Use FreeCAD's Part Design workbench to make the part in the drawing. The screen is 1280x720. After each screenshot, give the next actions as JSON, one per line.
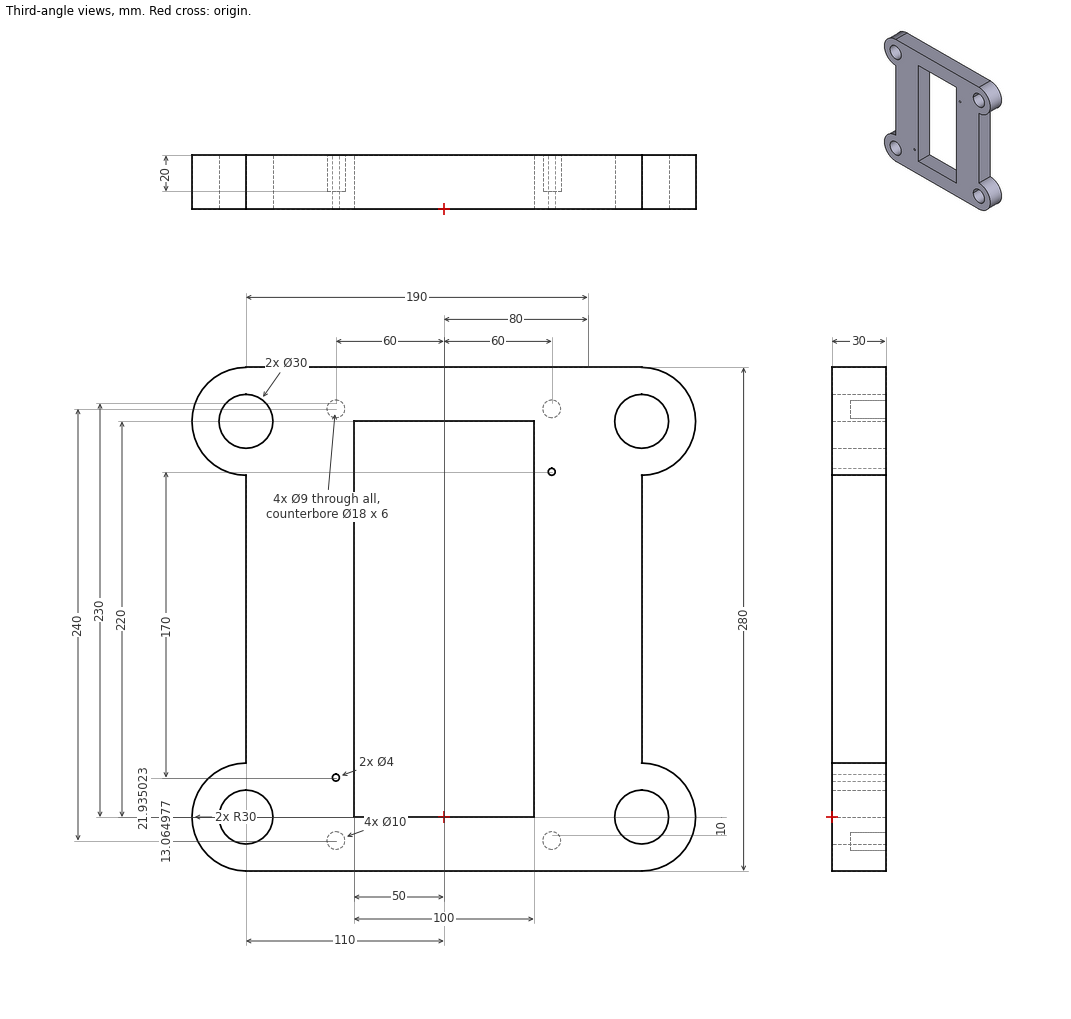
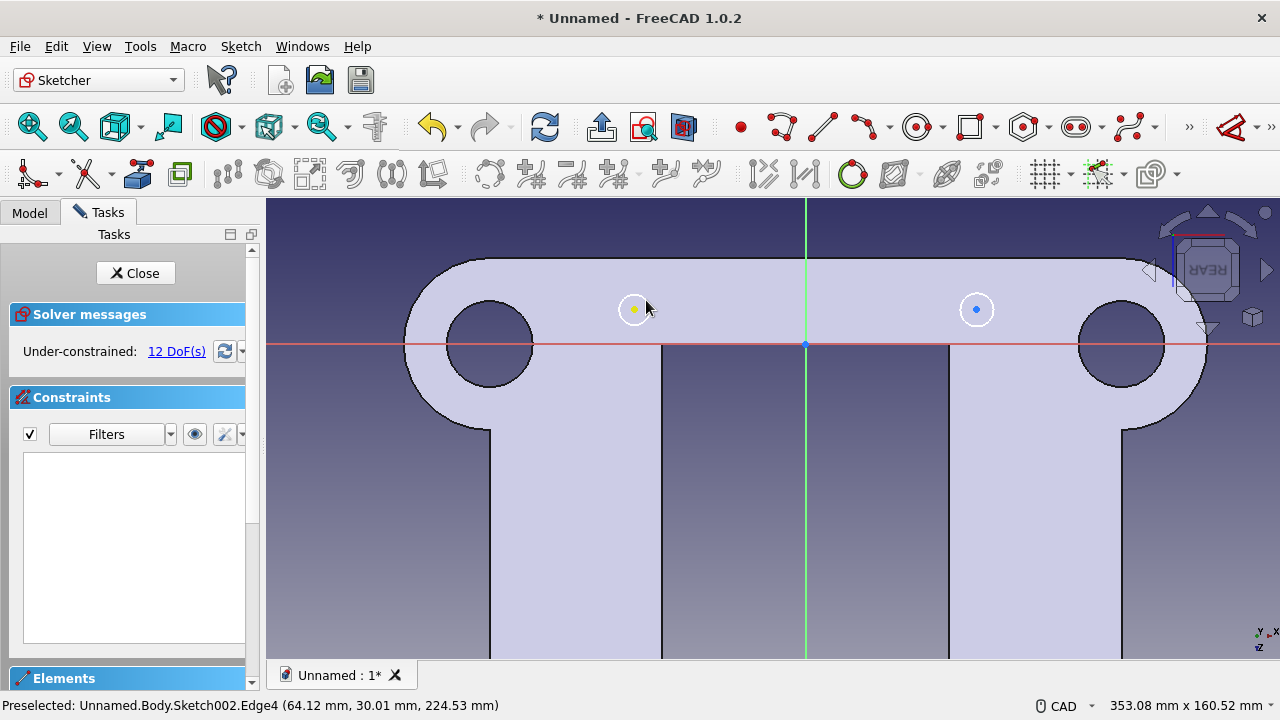
{"action": "left_click", "coordinate": [645, 299]}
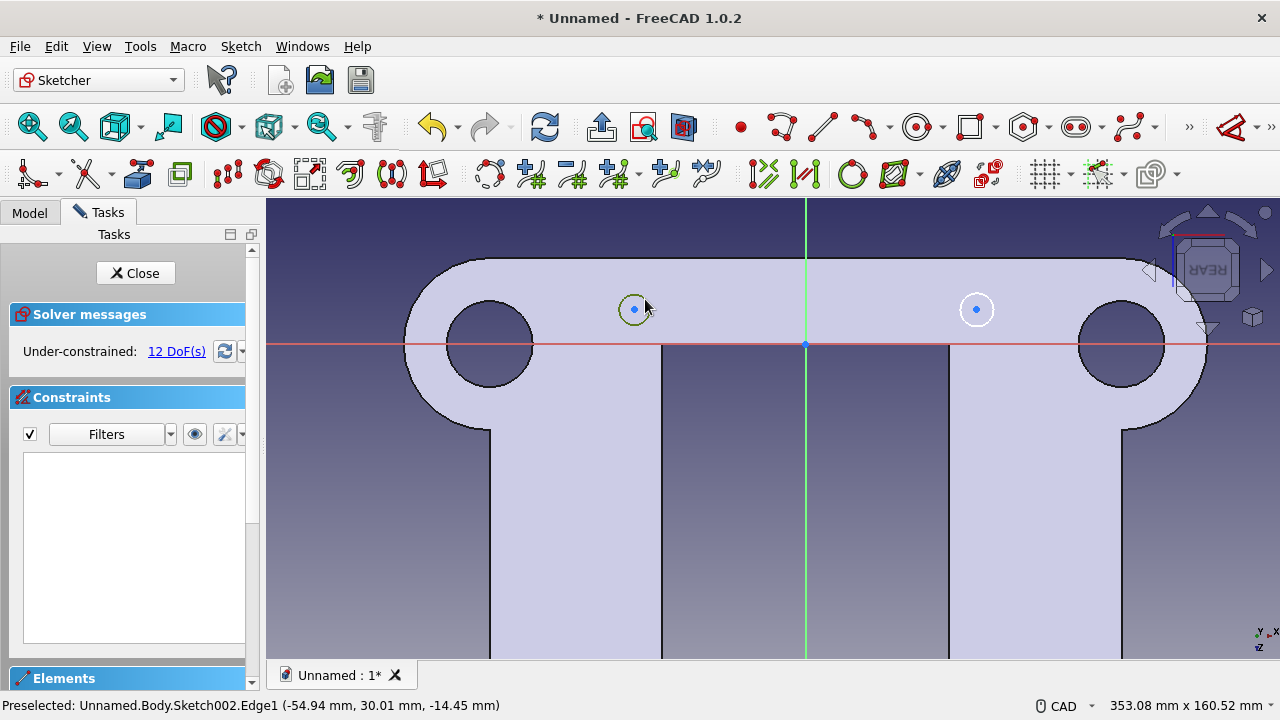
{"action": "scroll", "coordinate": [646, 299], "scroll_direction": "down", "scroll_amount": 5}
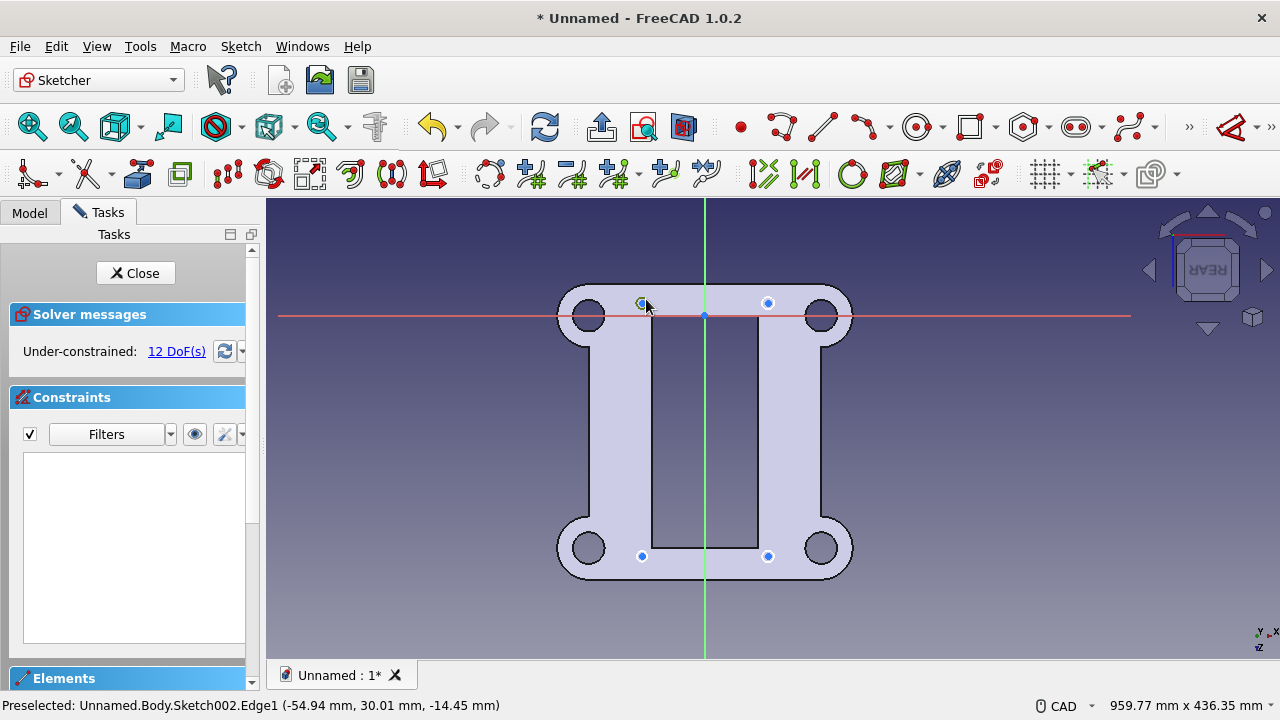
{"action": "scroll", "coordinate": [646, 553], "scroll_direction": "up", "scroll_amount": 5}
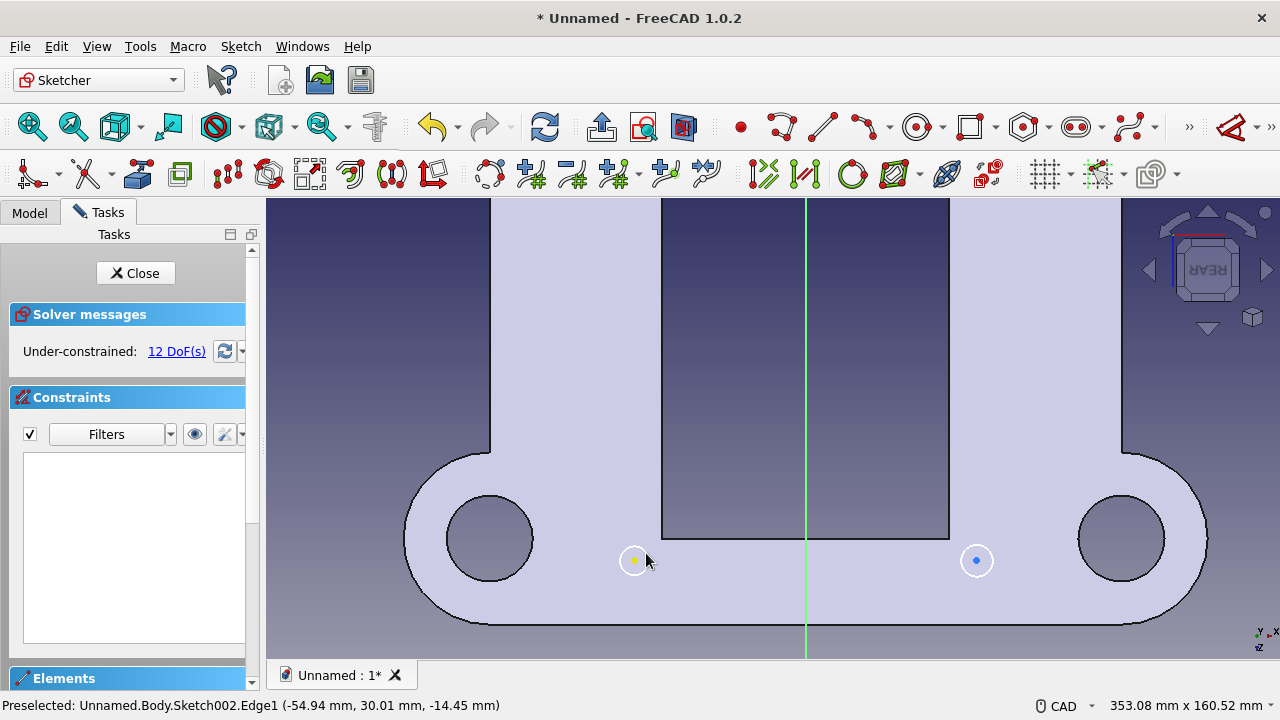
{"action": "left_click", "coordinate": [645, 551]}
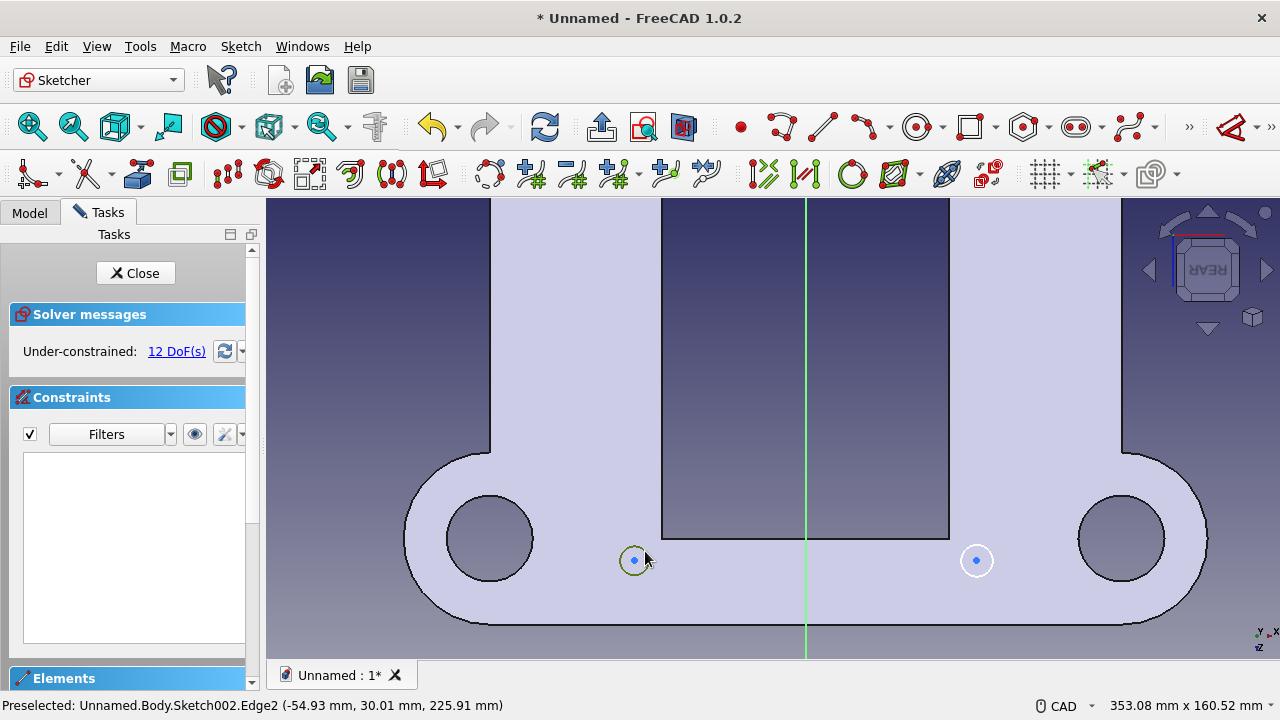
{"action": "scroll", "coordinate": [646, 553], "scroll_direction": "down", "scroll_amount": 5}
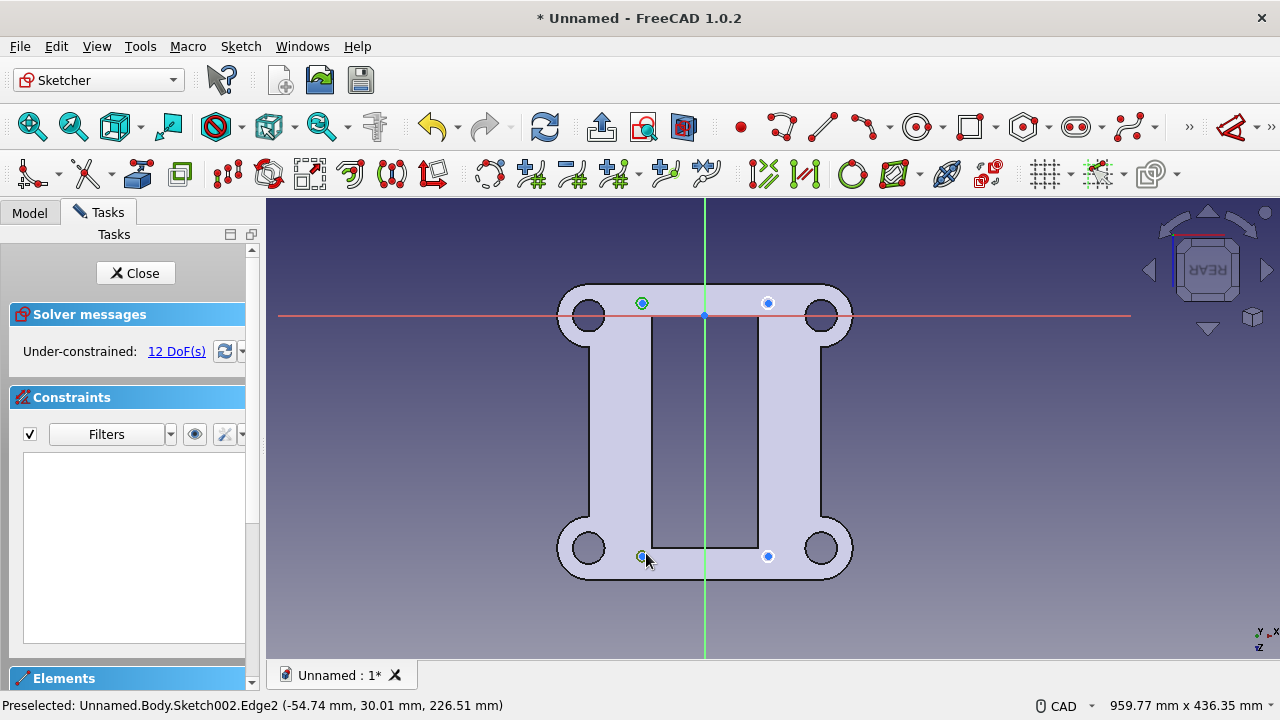
{"action": "scroll", "coordinate": [772, 299], "scroll_direction": "up", "scroll_amount": 5}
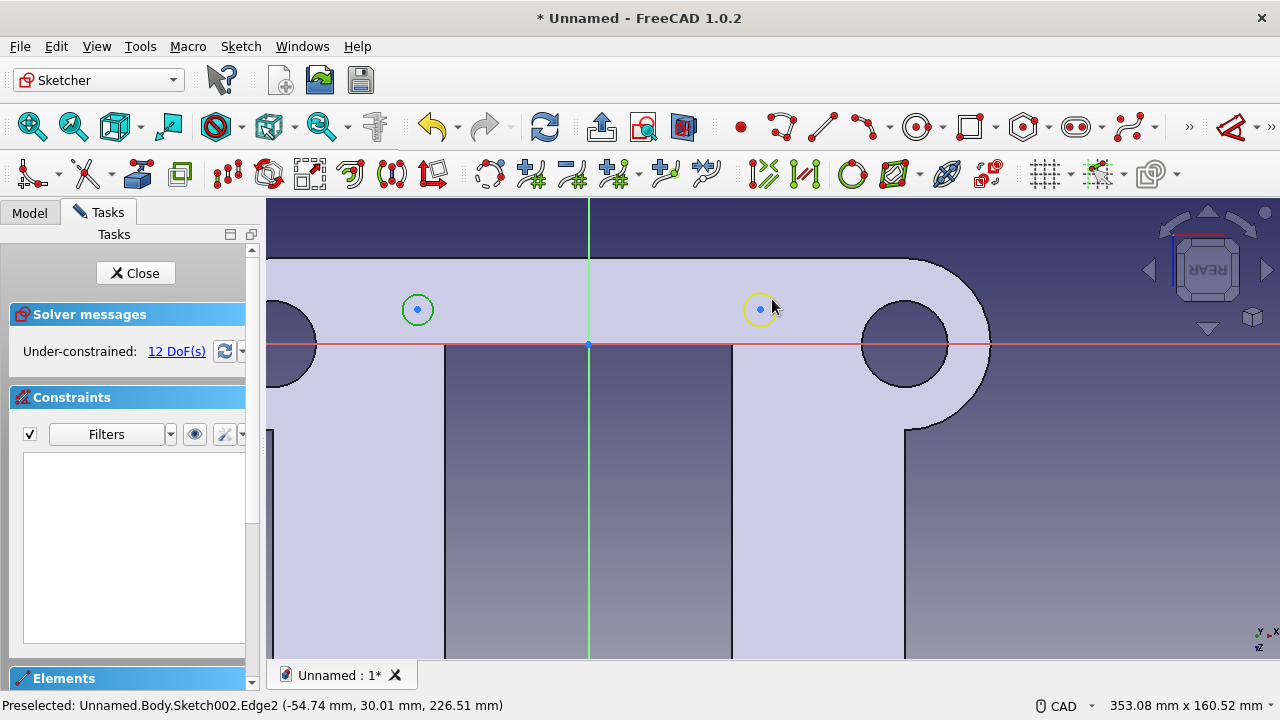
{"action": "left_click", "coordinate": [772, 298]}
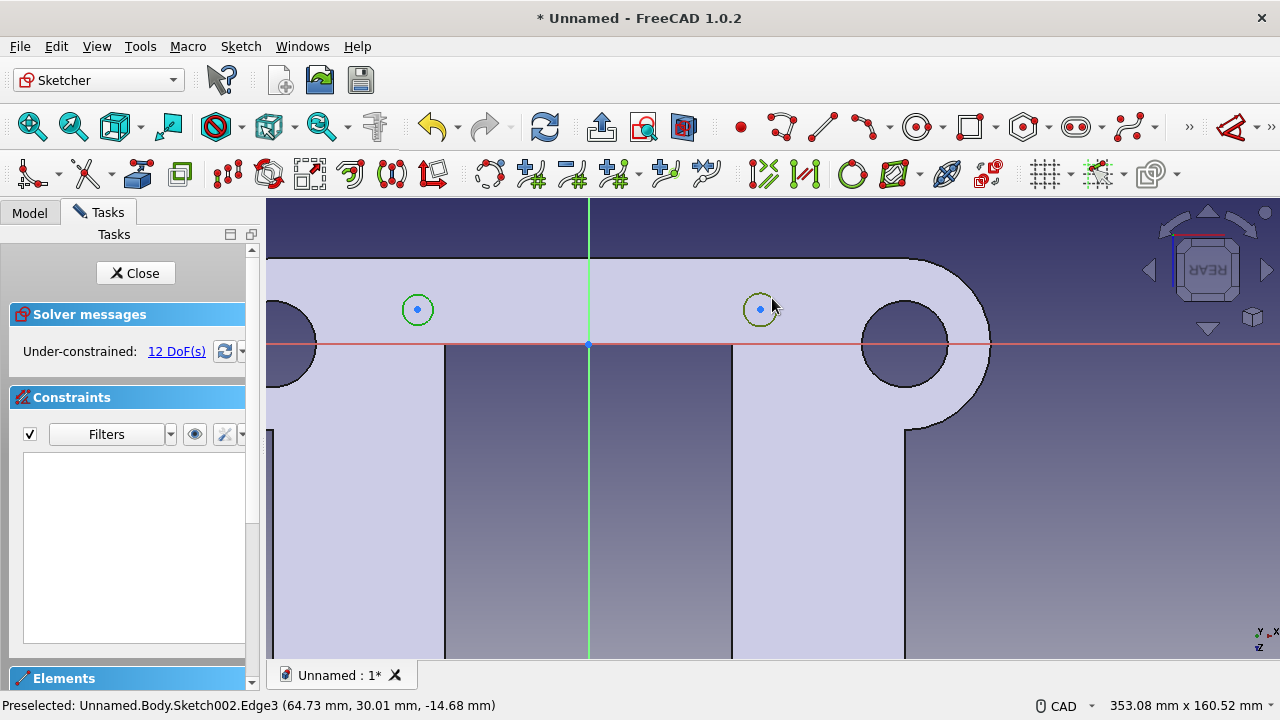
{"action": "scroll", "coordinate": [772, 299], "scroll_direction": "down", "scroll_amount": 5}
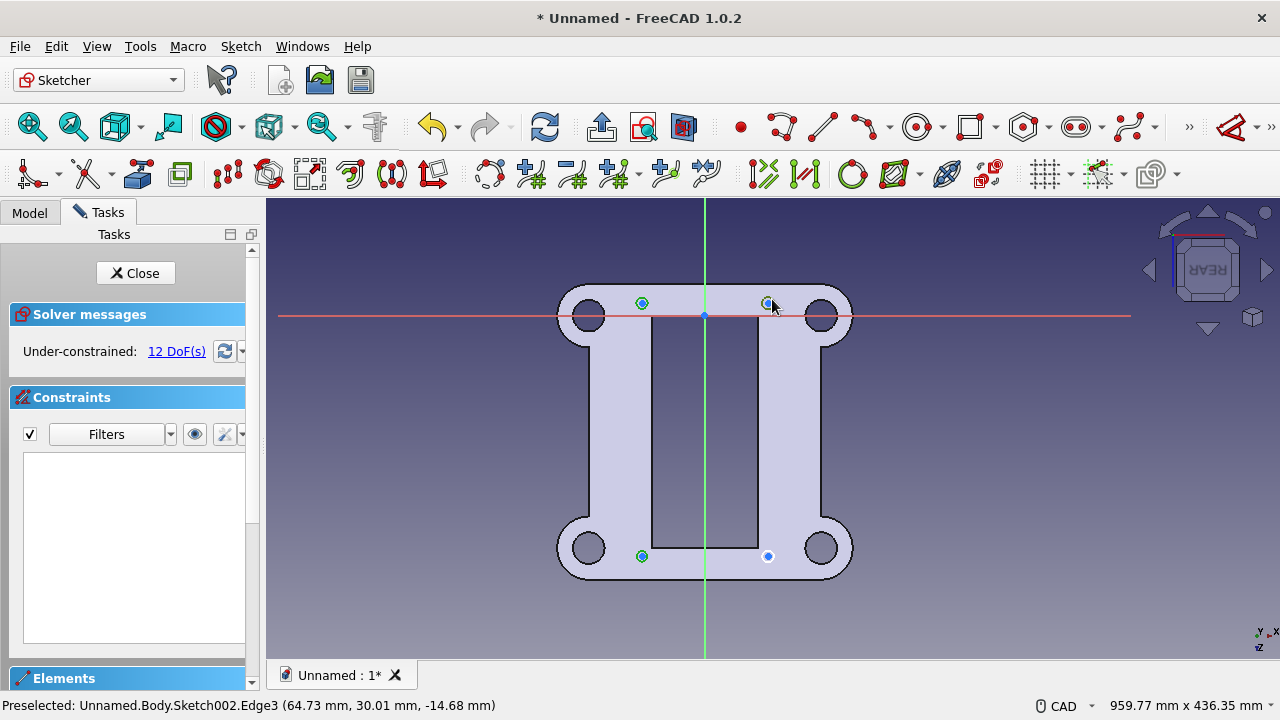
{"action": "scroll", "coordinate": [772, 552], "scroll_direction": "up", "scroll_amount": 5}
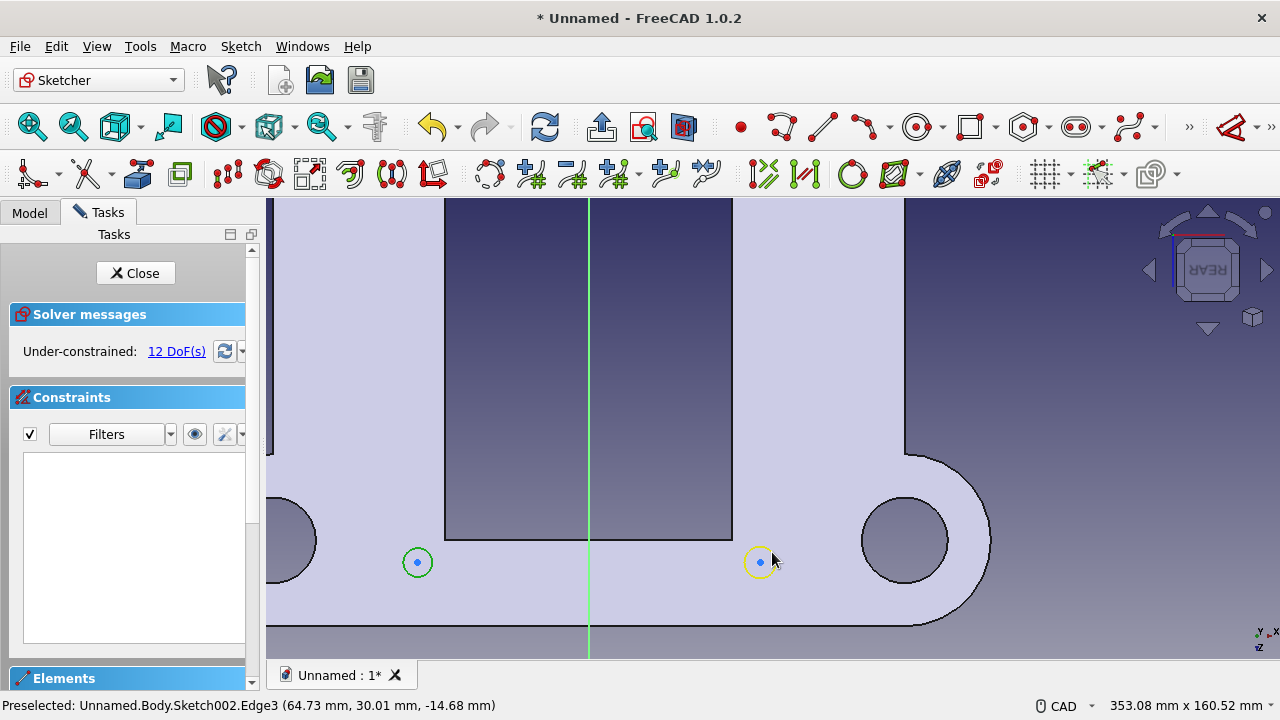
{"action": "left_click", "coordinate": [771, 551]}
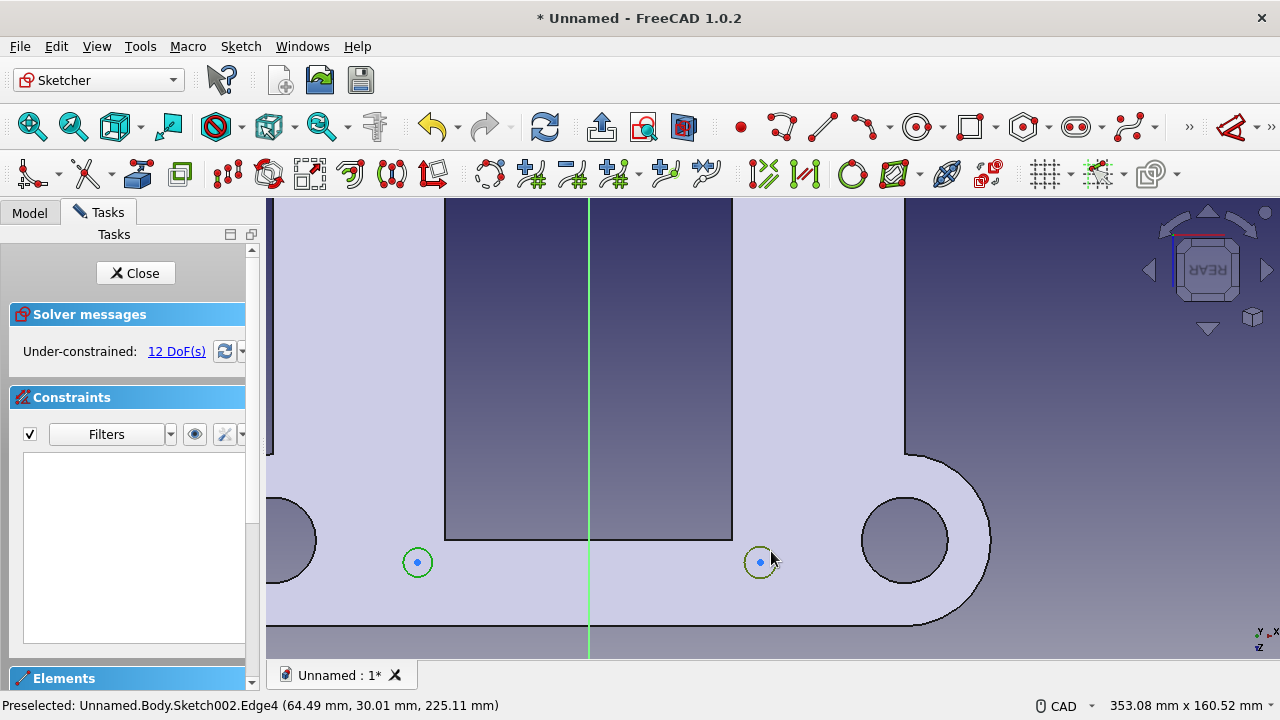
{"action": "key", "text": "e"}